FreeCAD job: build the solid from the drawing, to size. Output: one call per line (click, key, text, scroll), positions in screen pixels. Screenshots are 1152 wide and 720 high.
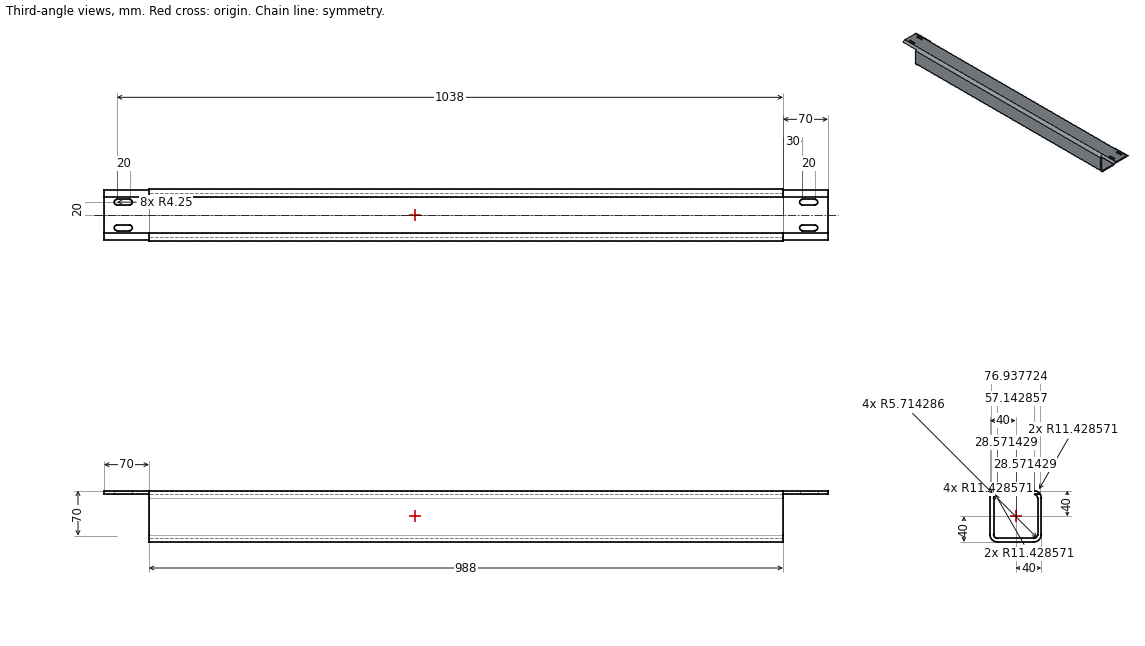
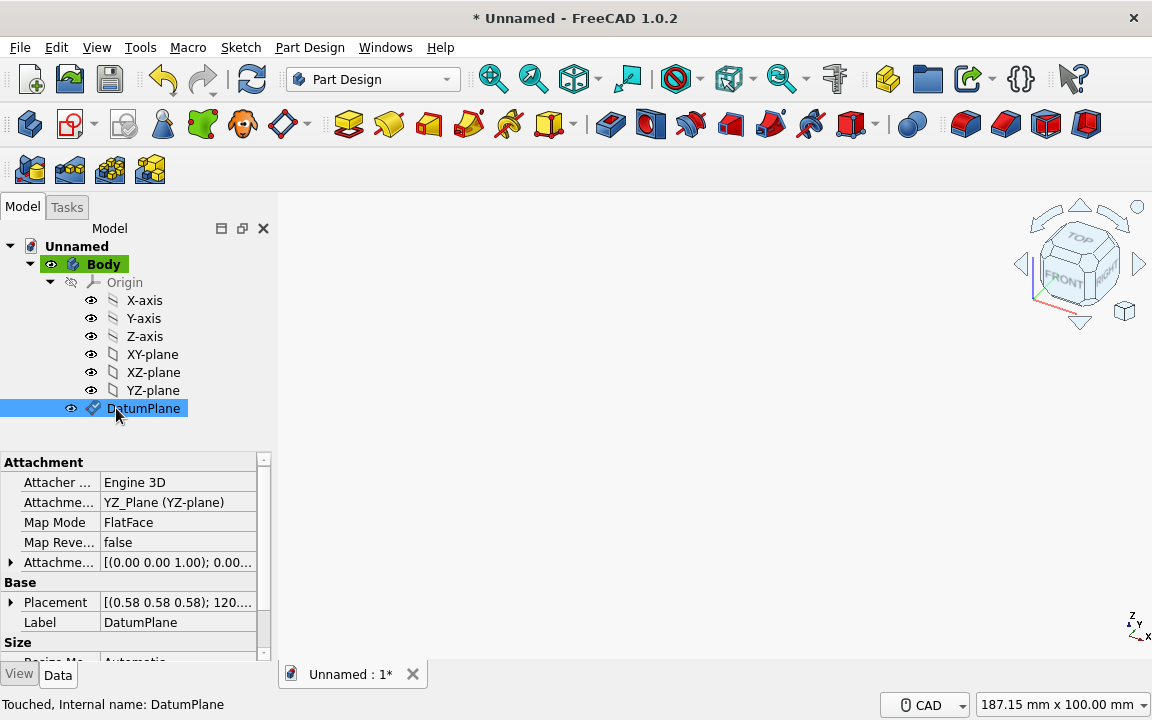
click(70, 124)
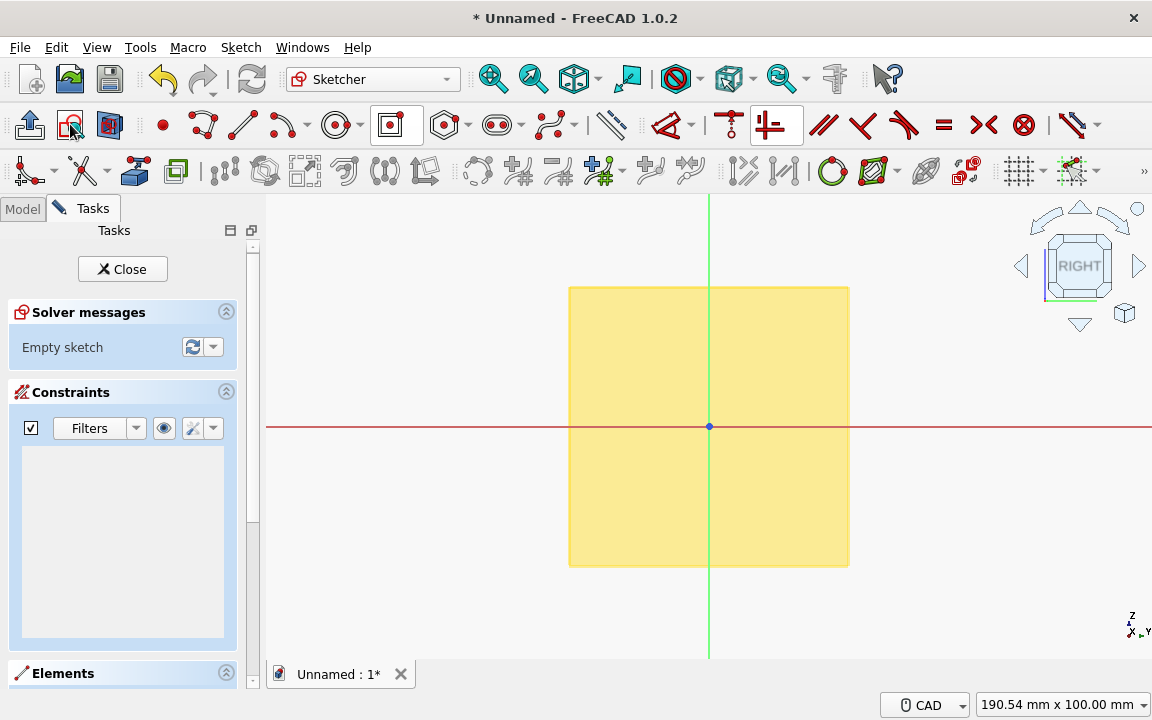
scroll(331, 427, down, 1)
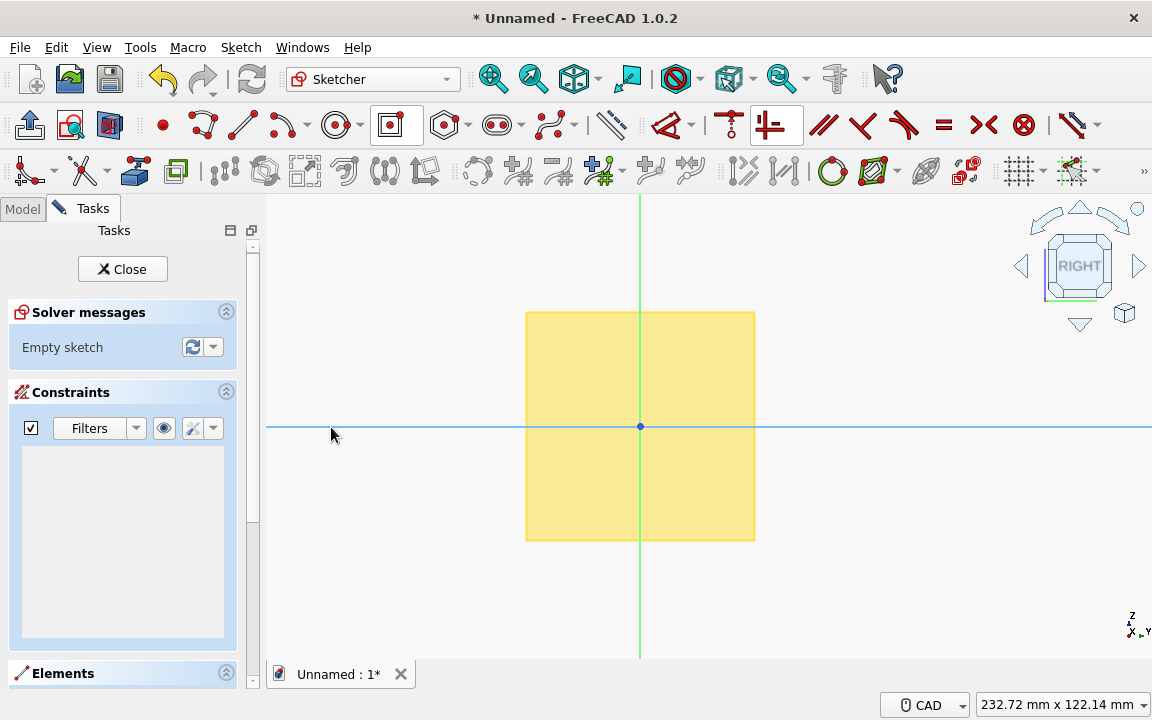
click(244, 126)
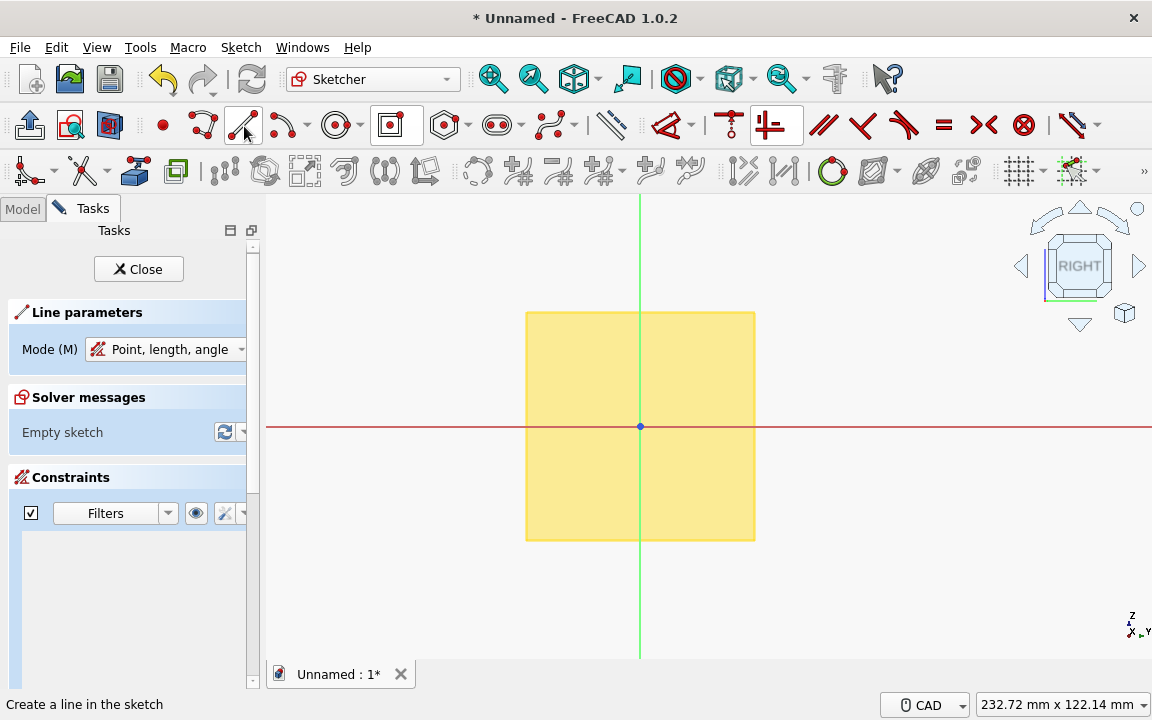
click(532, 579)
click(749, 579)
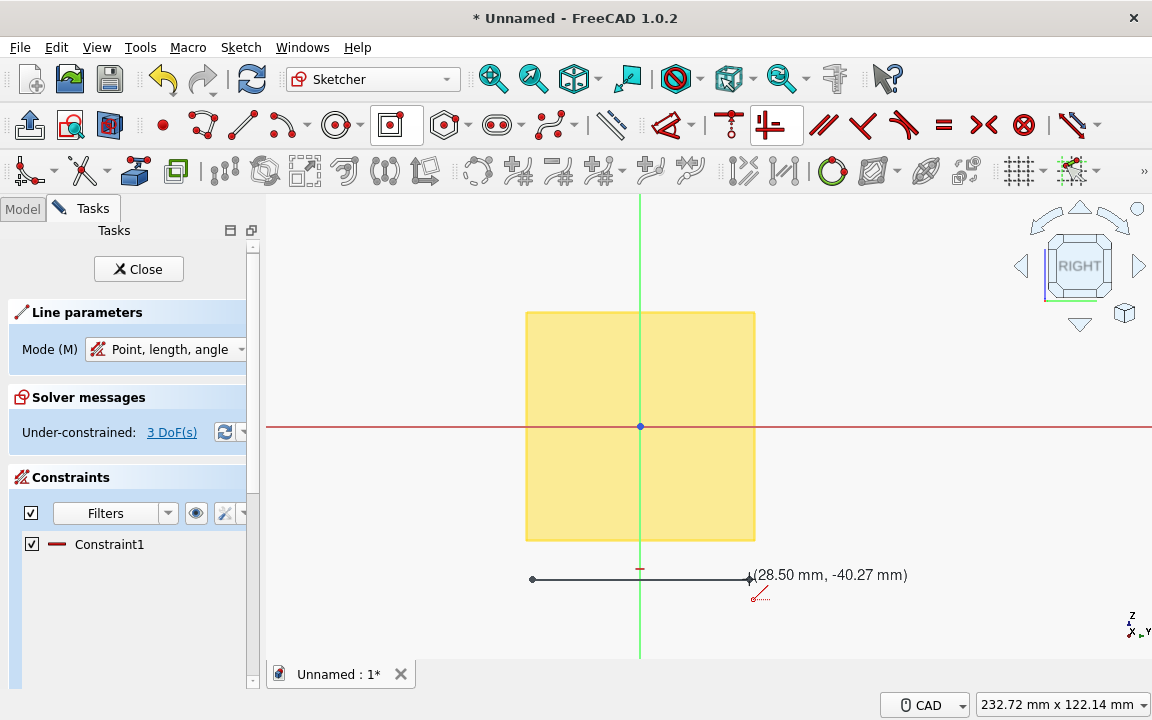
click(793, 535)
click(793, 318)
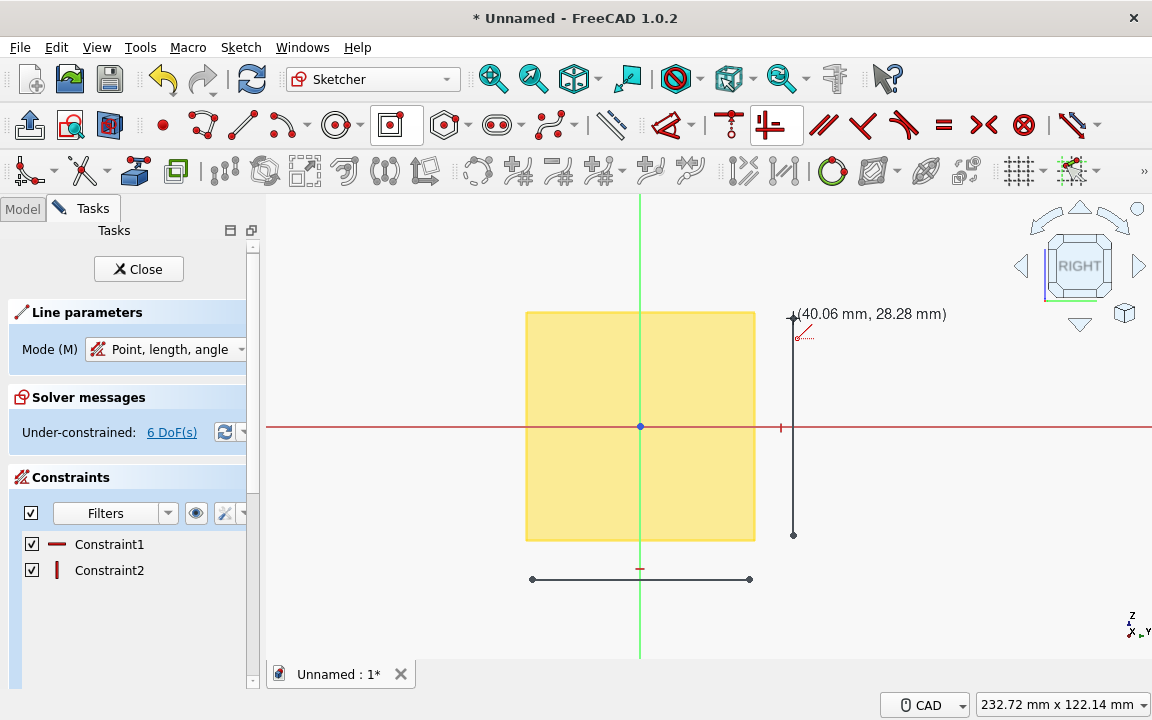
click(749, 274)
click(532, 274)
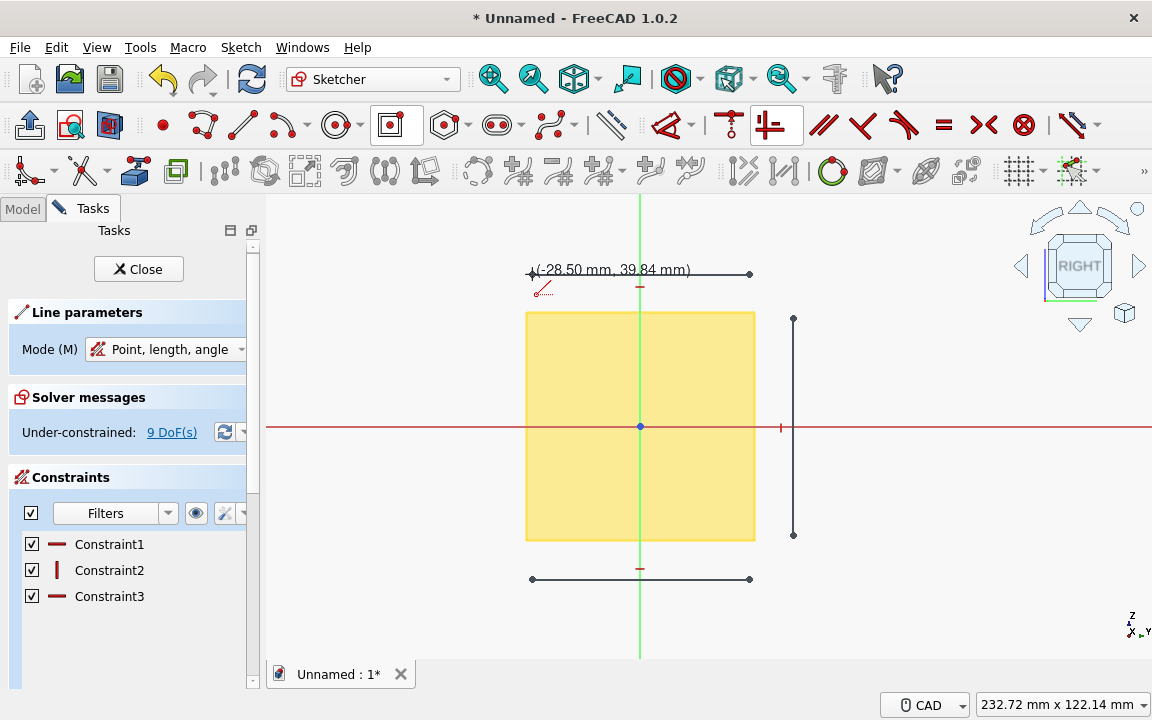
click(488, 318)
click(488, 535)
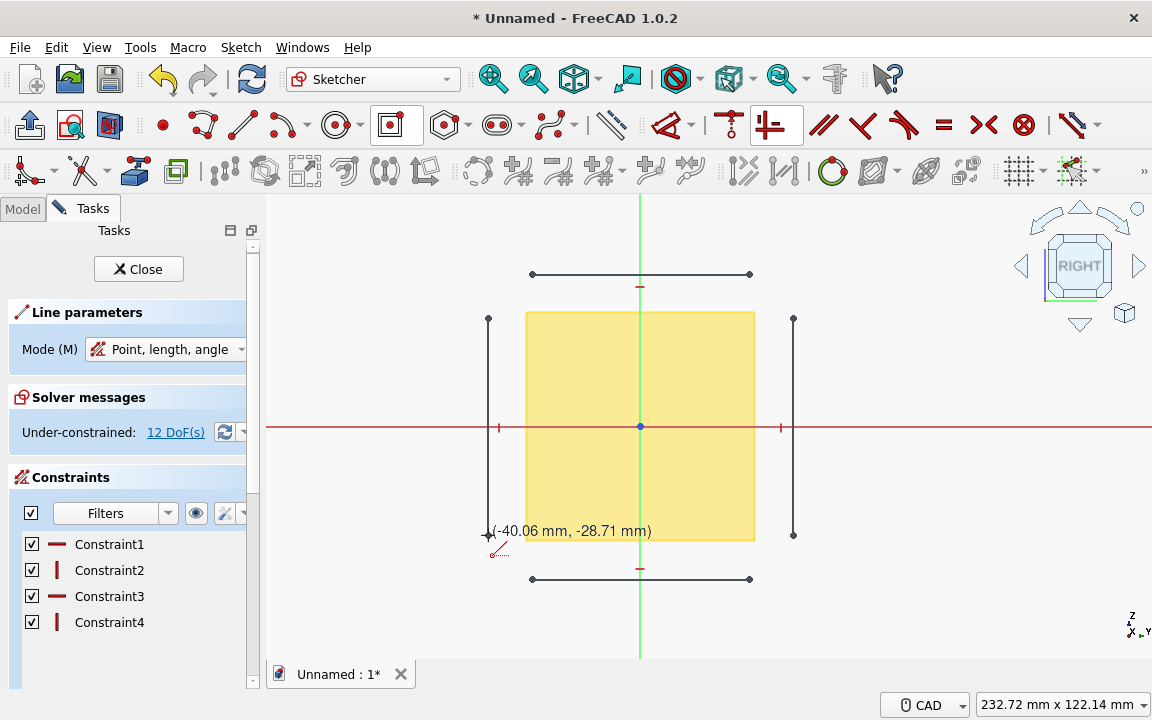
key(g)
key(3)
key(a)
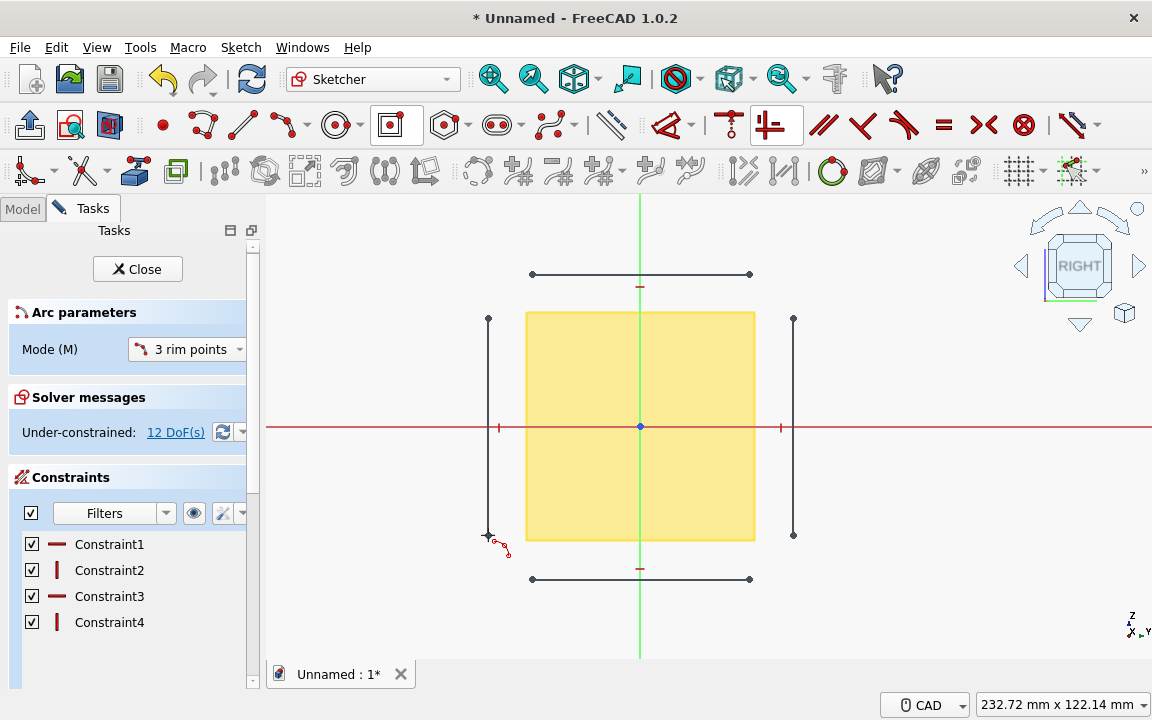
click(749, 580)
click(793, 536)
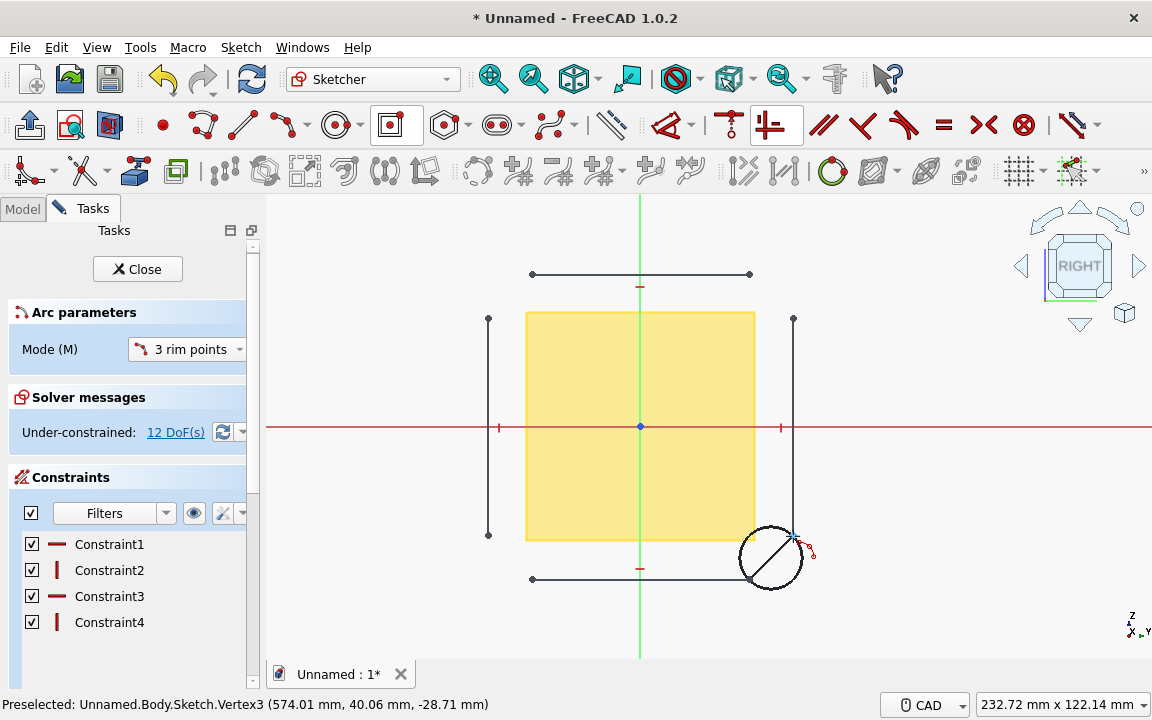
scroll(780, 566, up, 2)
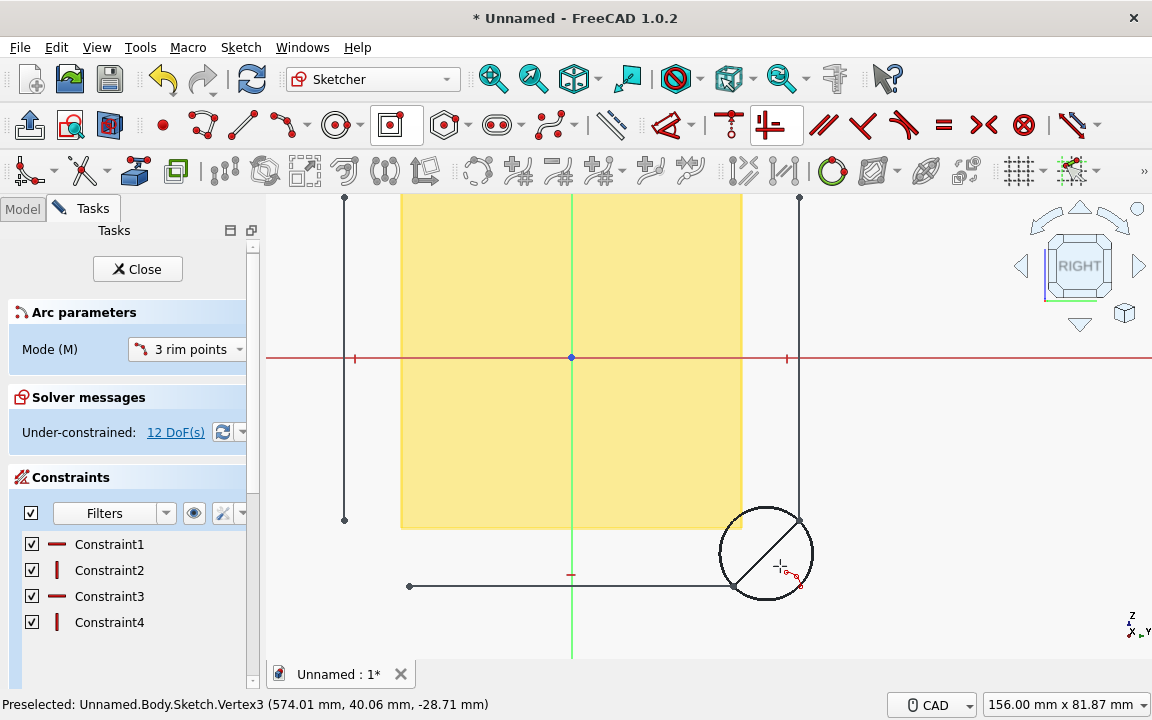
click(780, 566)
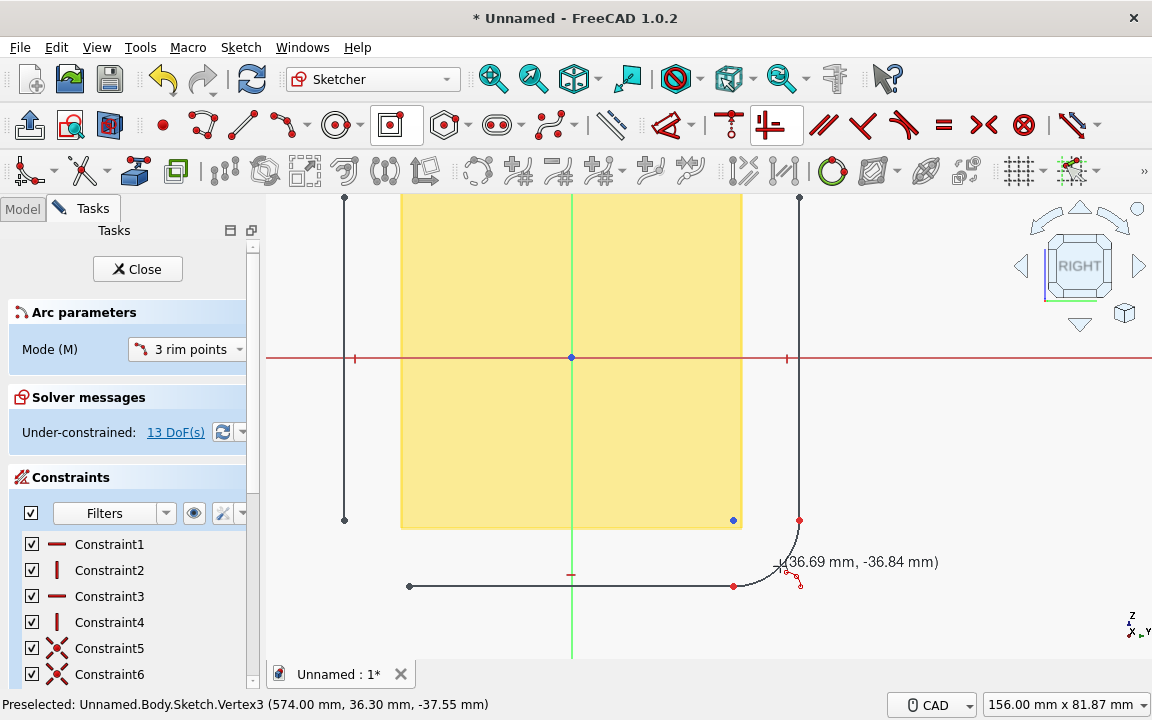
scroll(781, 566, down, 2)